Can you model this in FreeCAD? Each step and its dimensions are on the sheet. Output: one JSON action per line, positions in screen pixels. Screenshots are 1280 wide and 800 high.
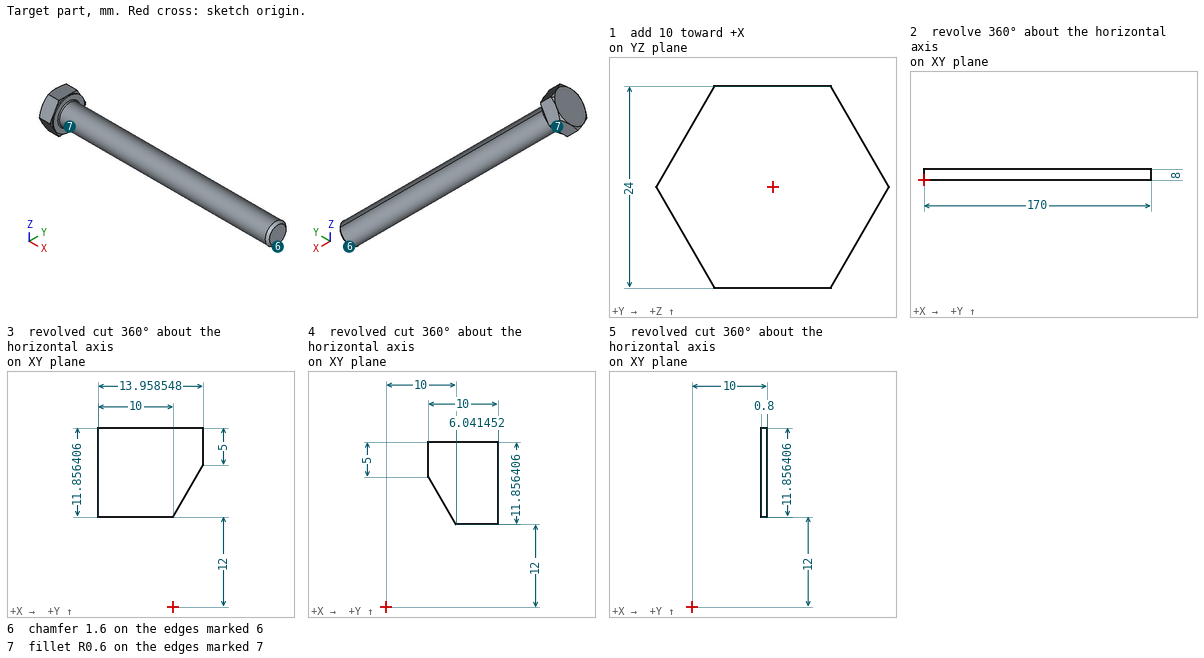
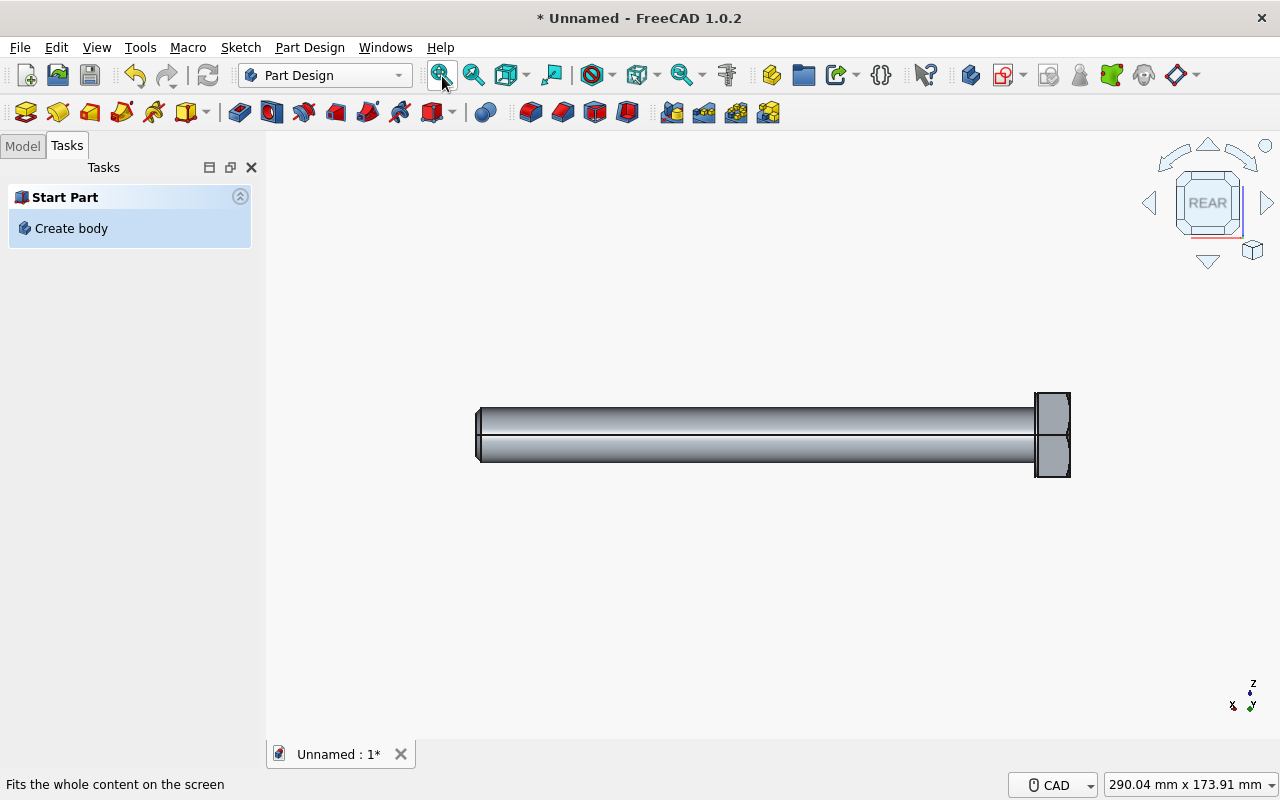
{"action": "key", "text": "6"}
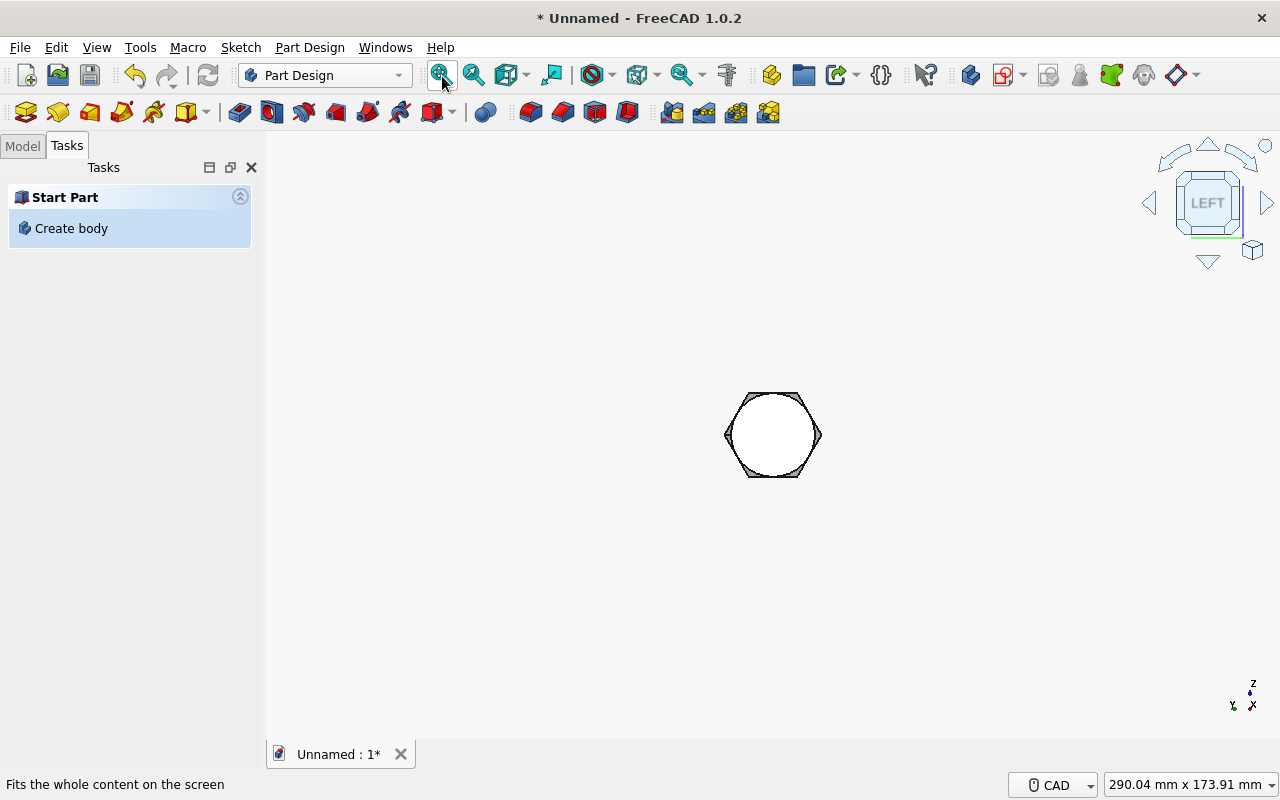
{"action": "left_click", "coordinate": [442, 76]}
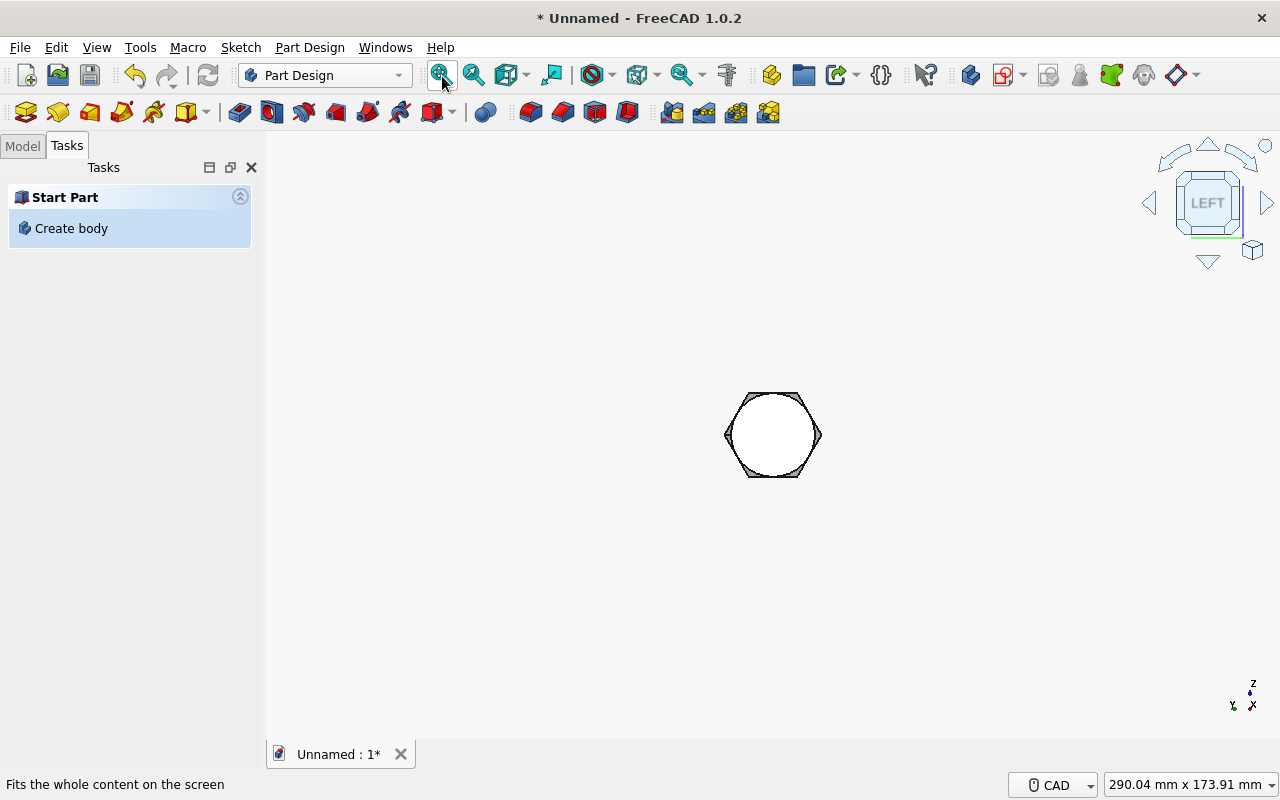
{"action": "key", "text": "v 3"}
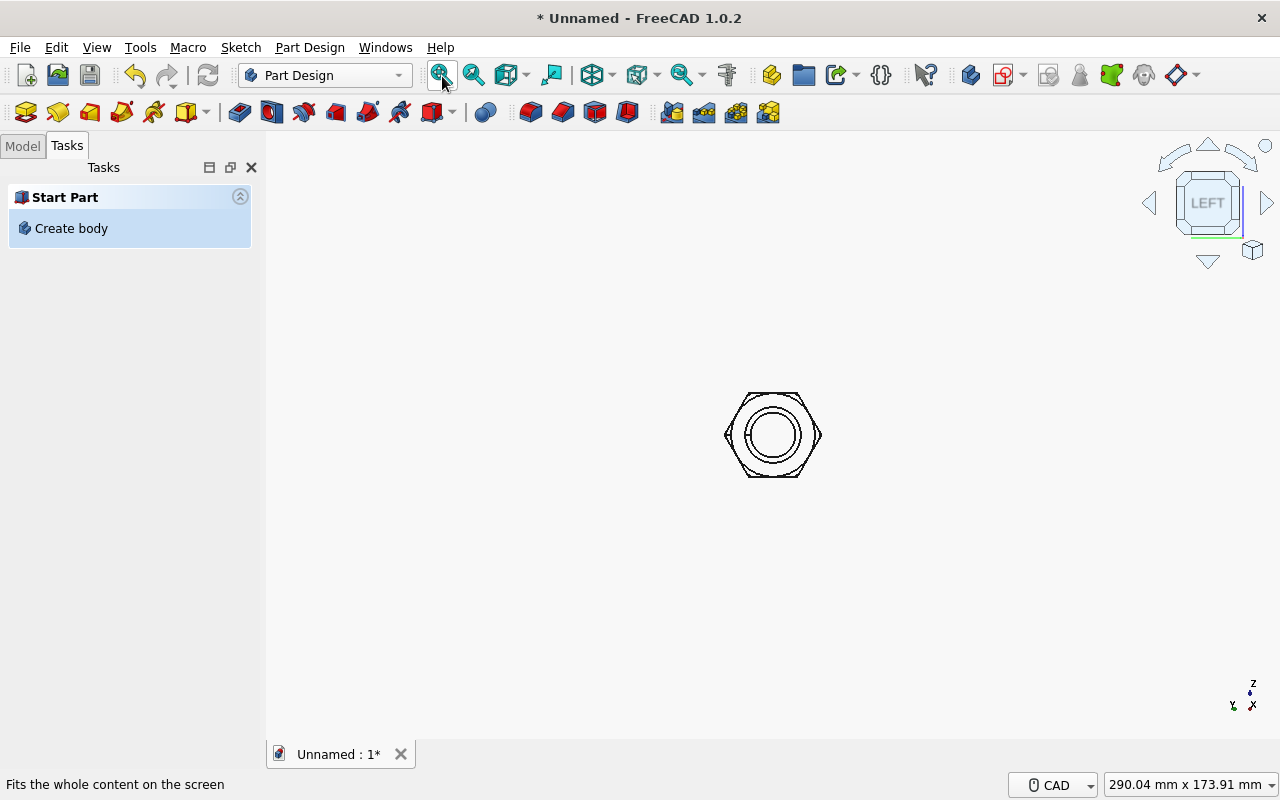
{"action": "key", "text": "0"}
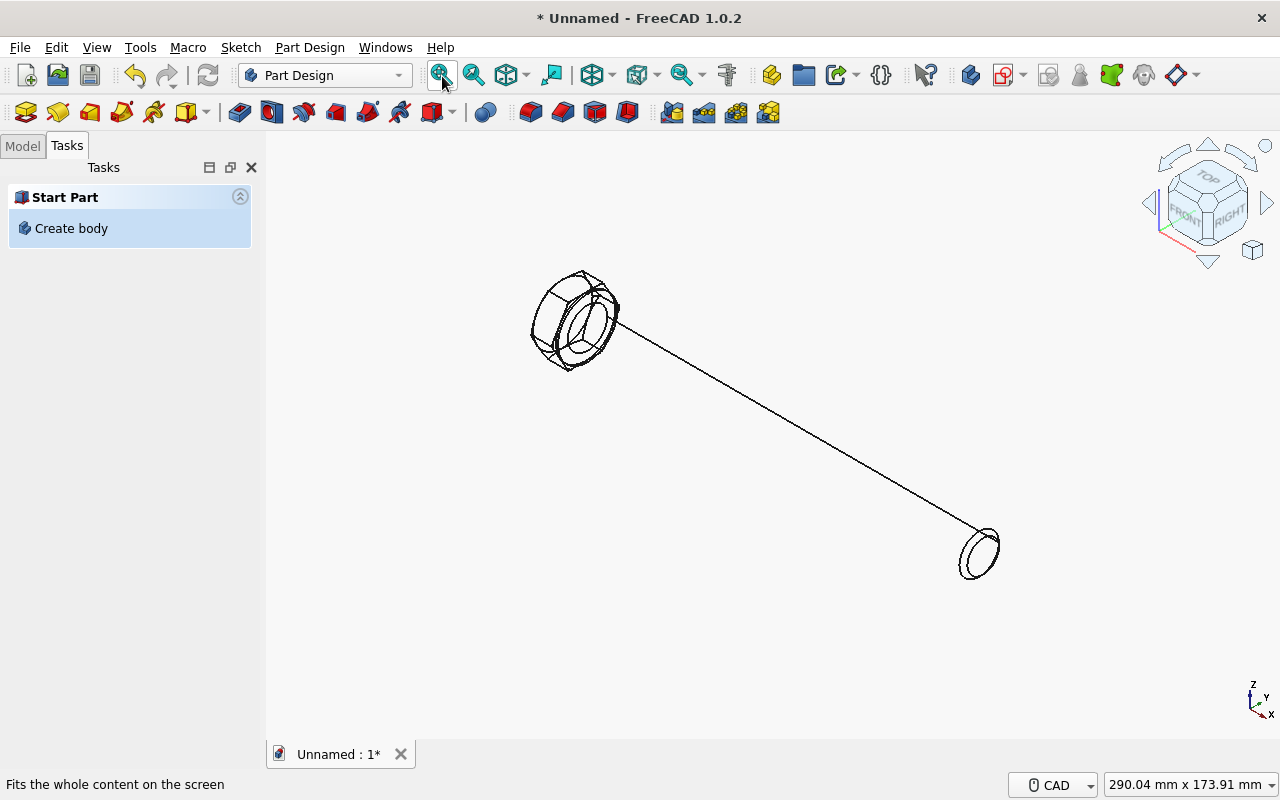
{"action": "left_click", "coordinate": [568, 338]}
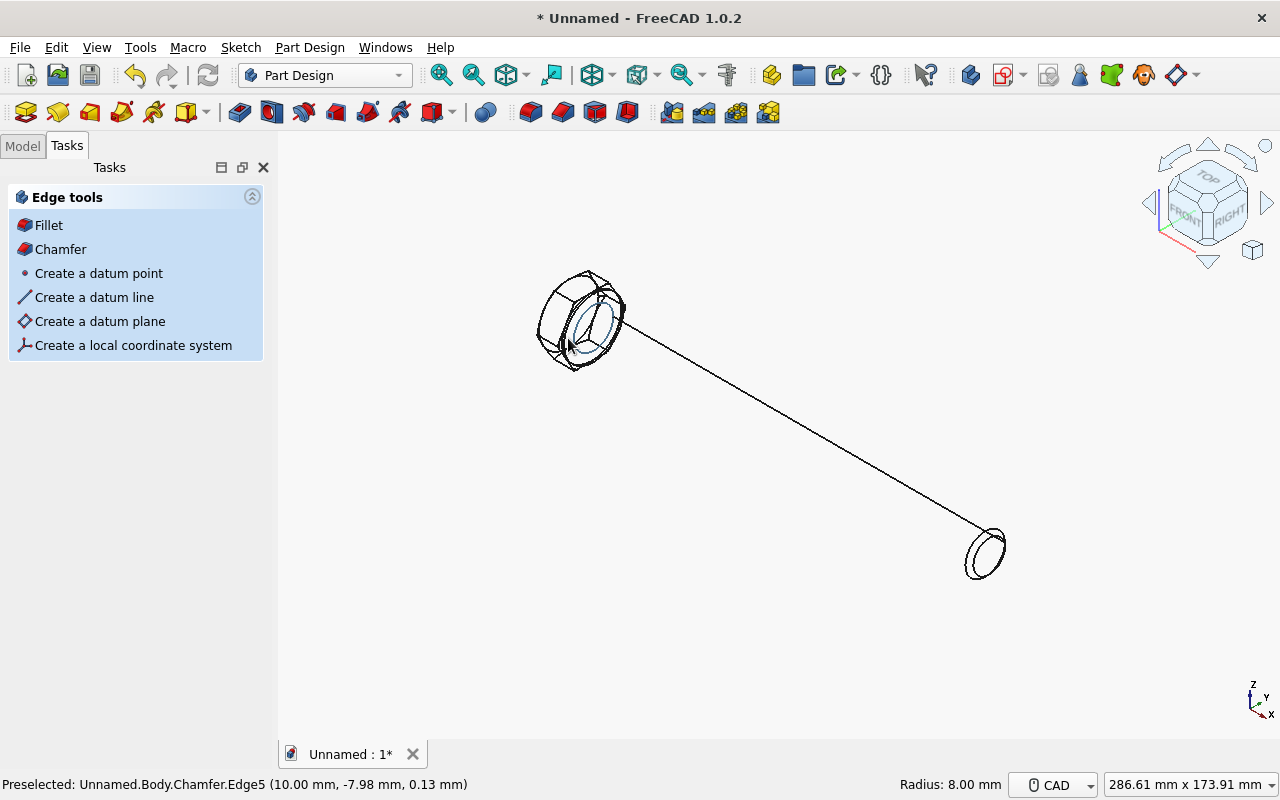
{"action": "key", "text": "v 1"}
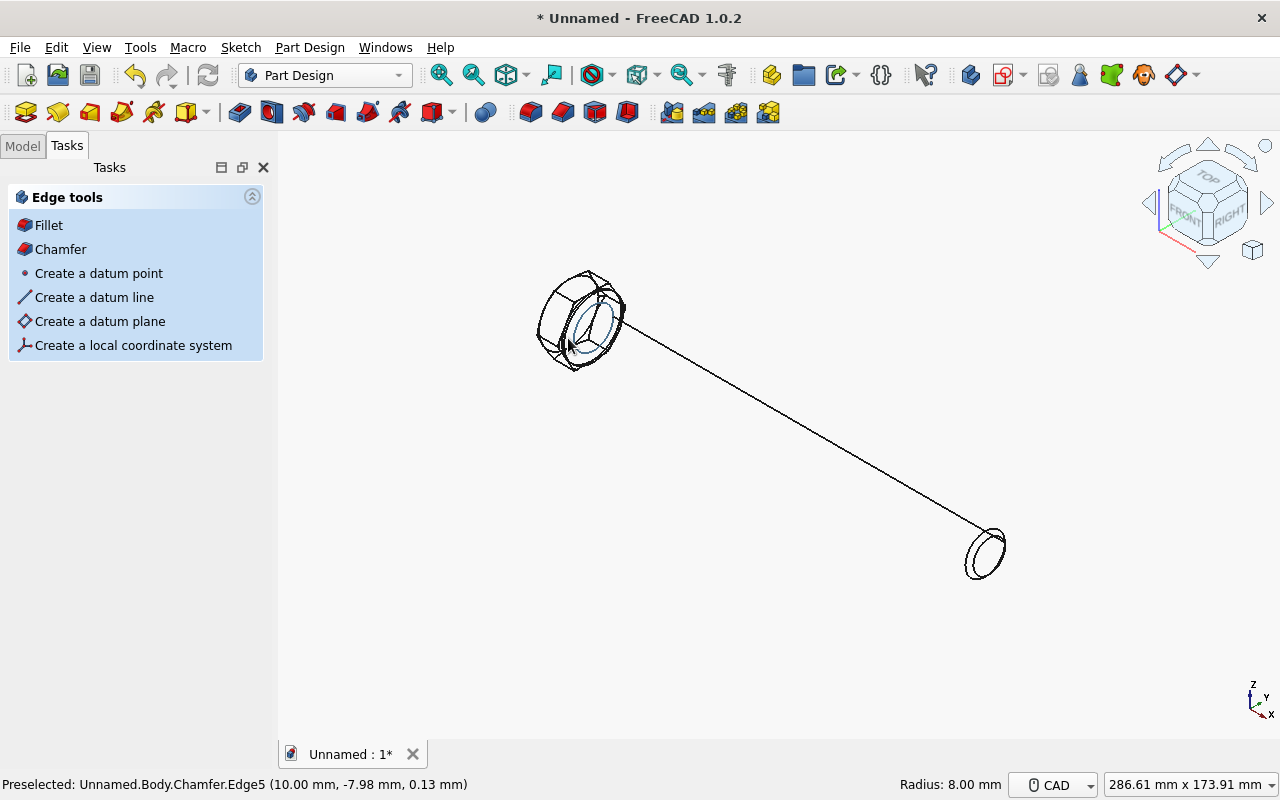
{"action": "left_click", "coordinate": [532, 112]}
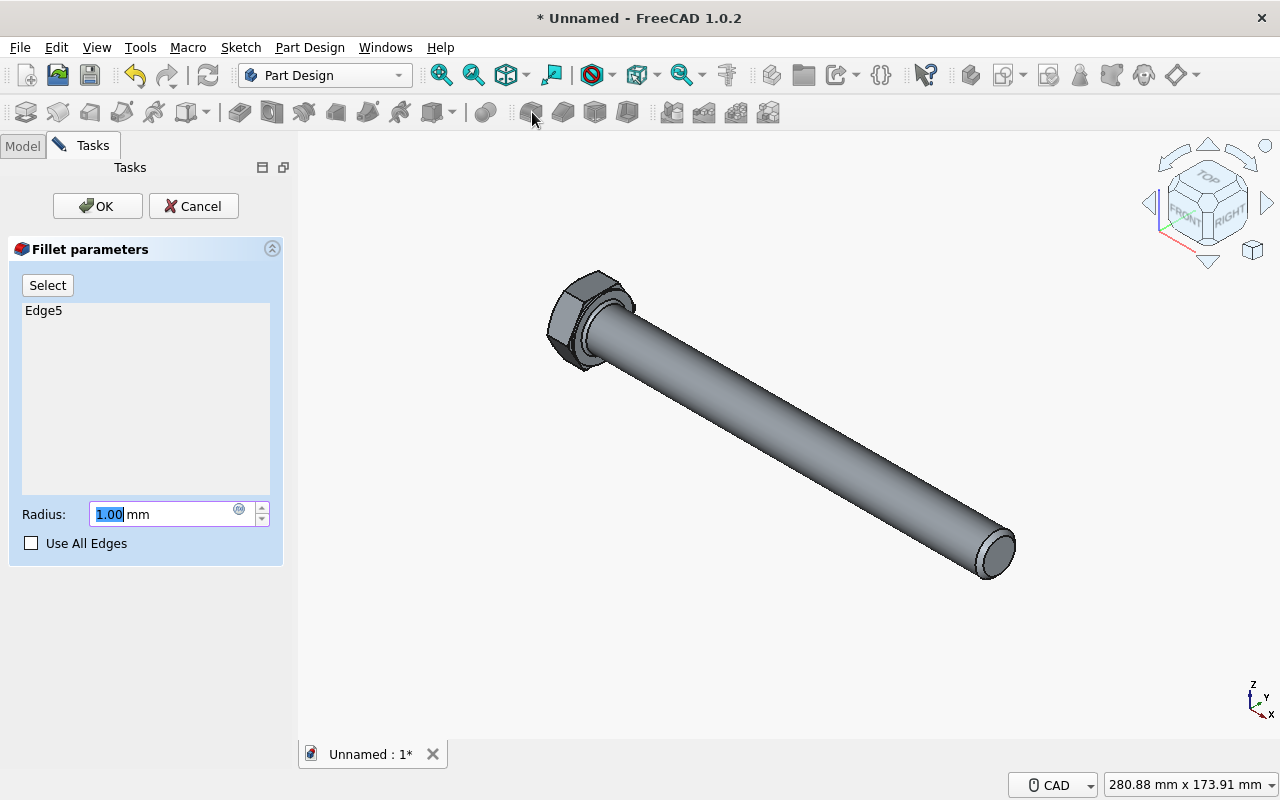
{"action": "type", "text": "0.6"}
{"action": "key", "text": "Tab"}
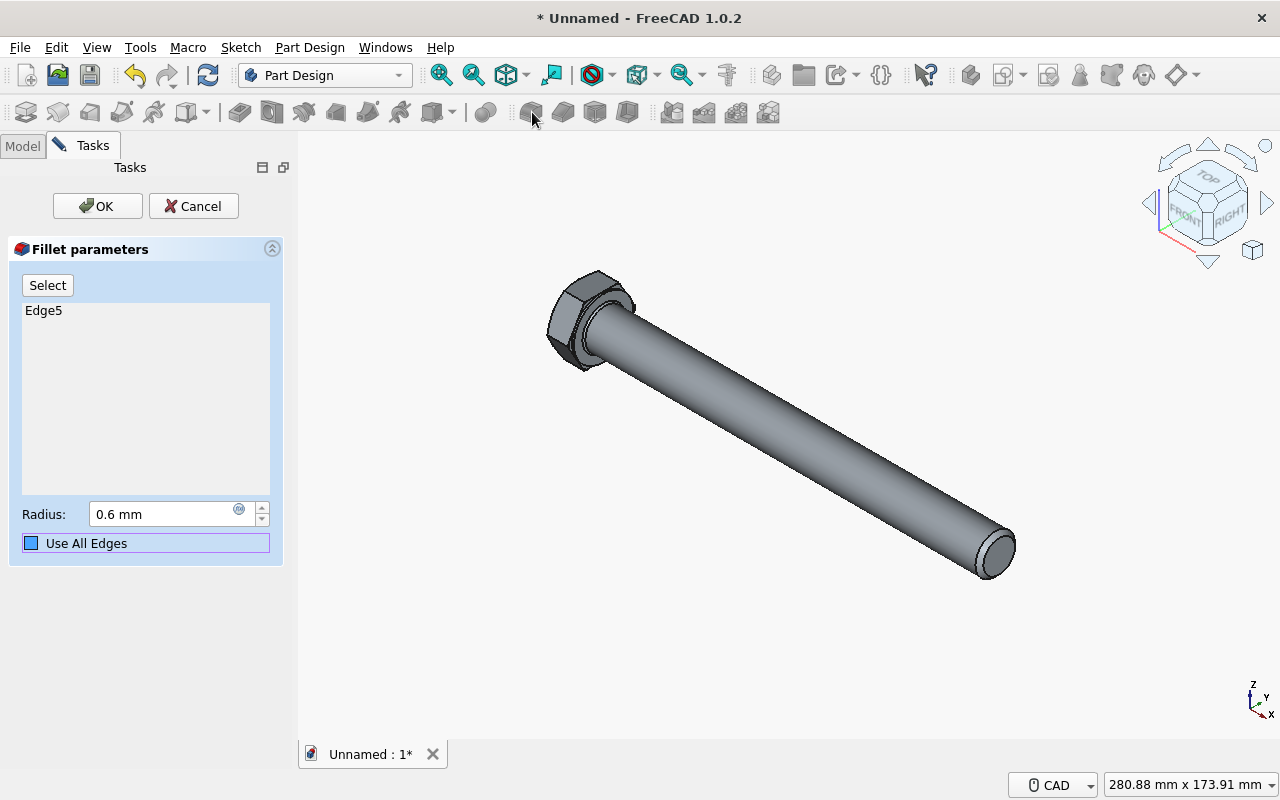
{"action": "left_click", "coordinate": [98, 206]}